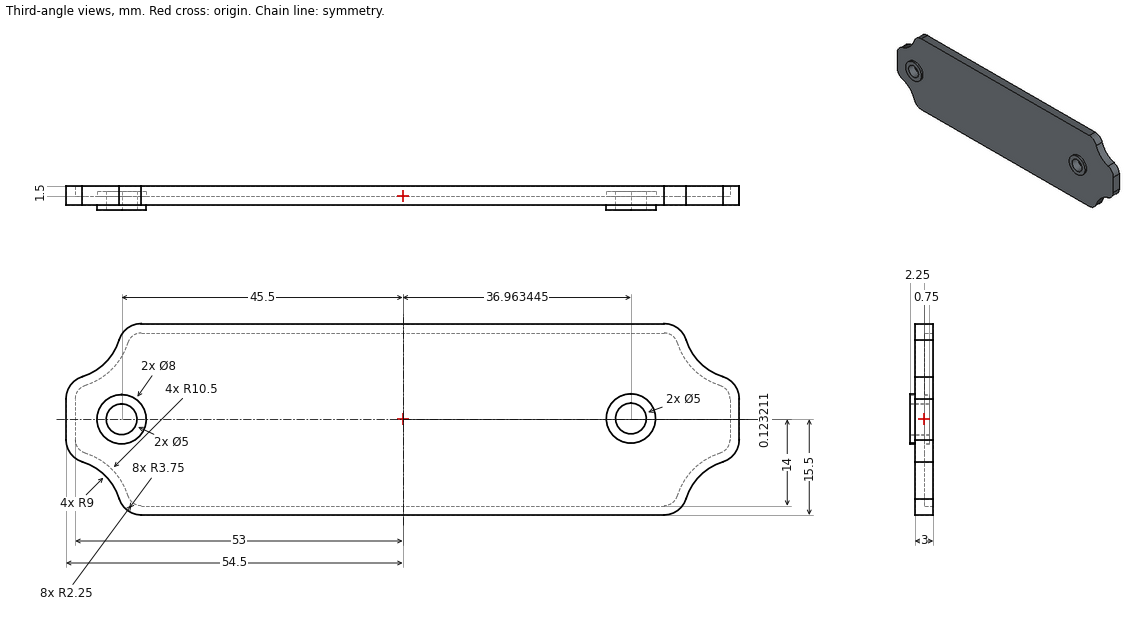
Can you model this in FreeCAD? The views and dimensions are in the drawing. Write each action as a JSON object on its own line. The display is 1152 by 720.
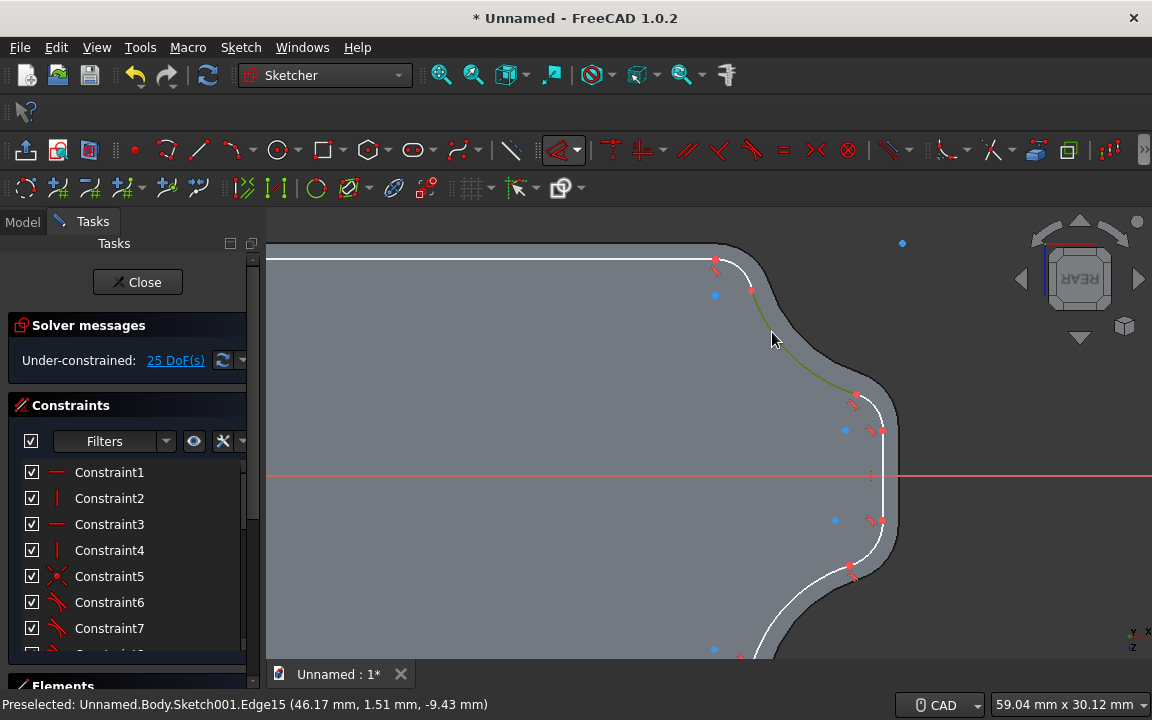
{"action": "left_click", "coordinate": [747, 276]}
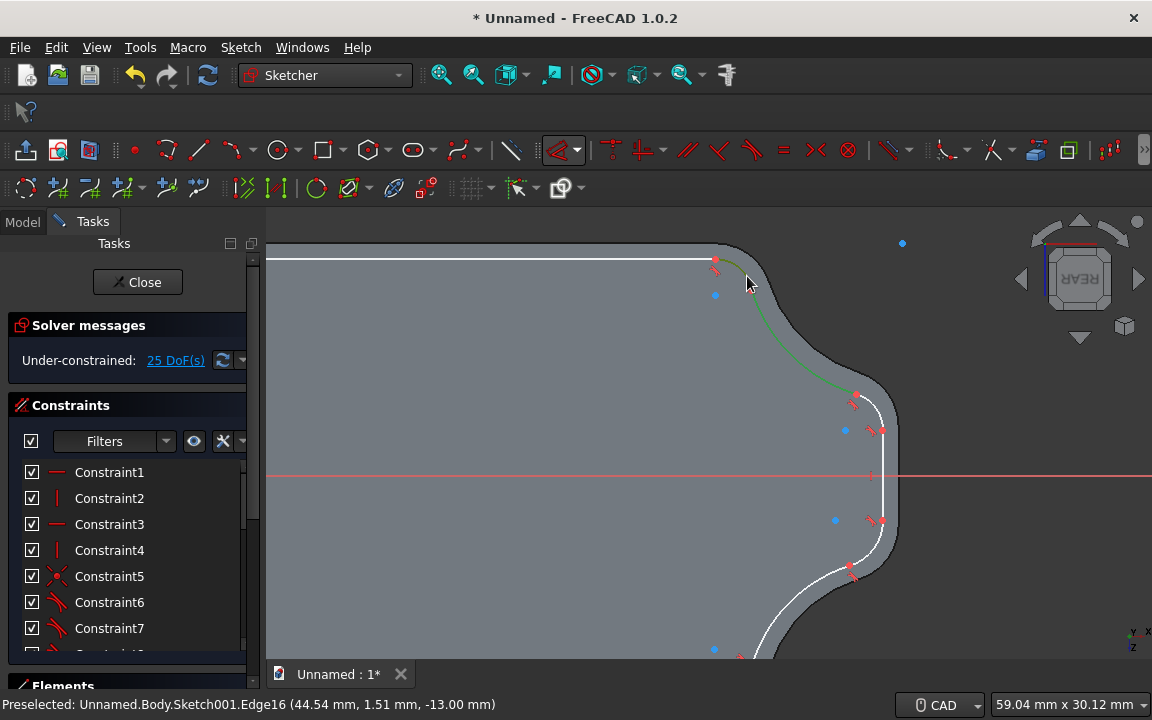
{"action": "left_click", "coordinate": [752, 150]}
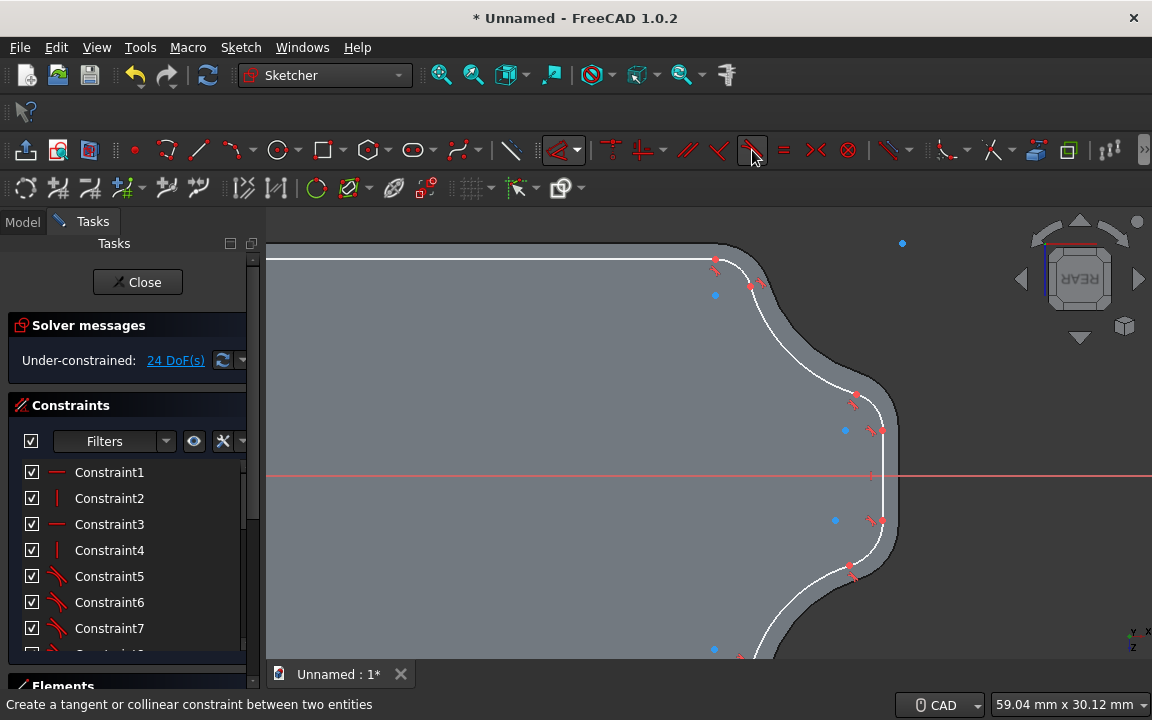
{"action": "scroll", "coordinate": [882, 415], "scroll_direction": "down", "scroll_amount": 6}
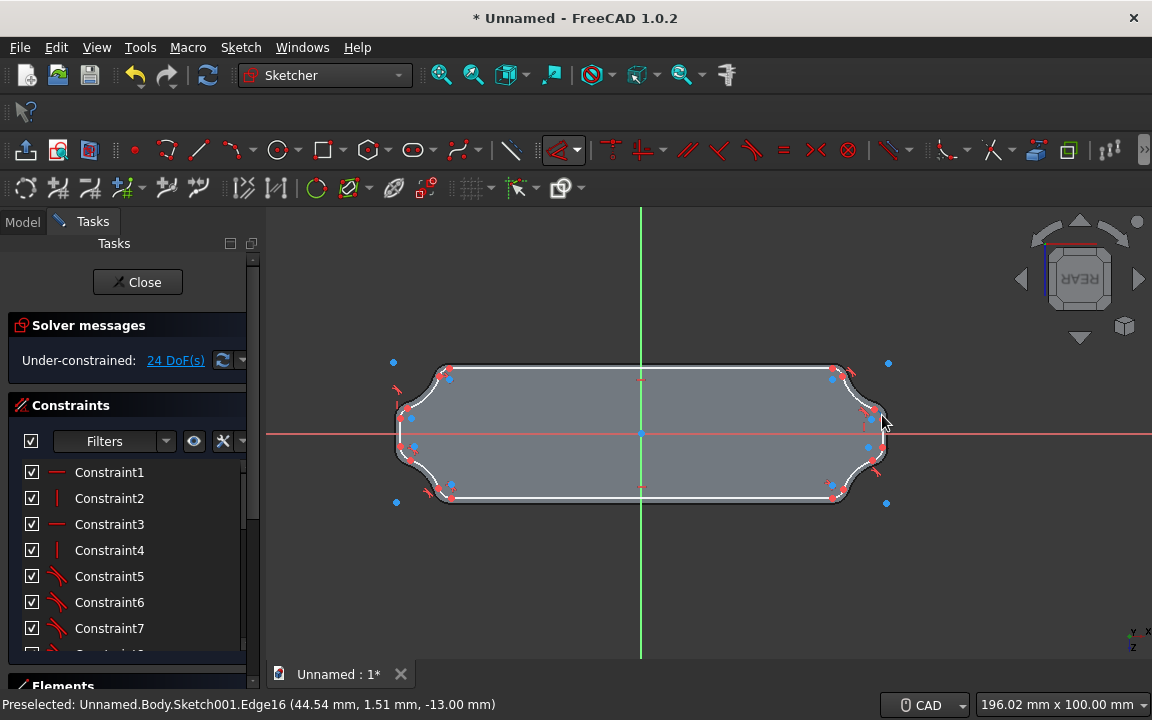
{"action": "scroll", "coordinate": [446, 369], "scroll_direction": "up", "scroll_amount": 7}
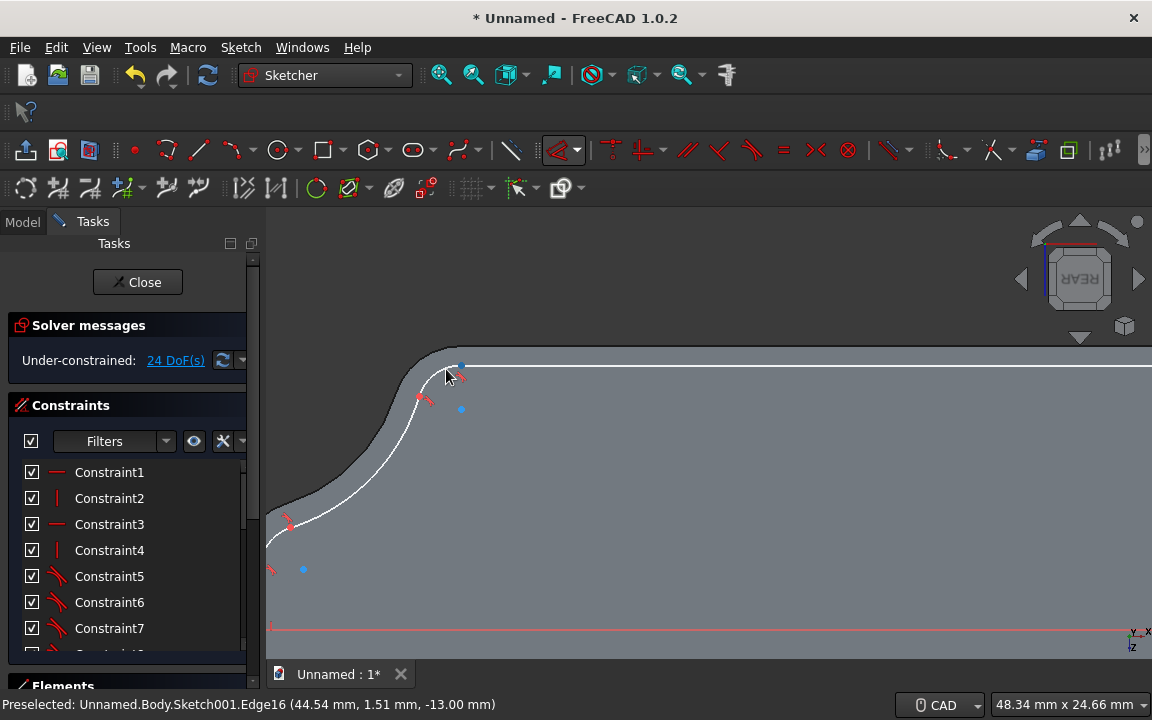
{"action": "left_click", "coordinate": [445, 369]}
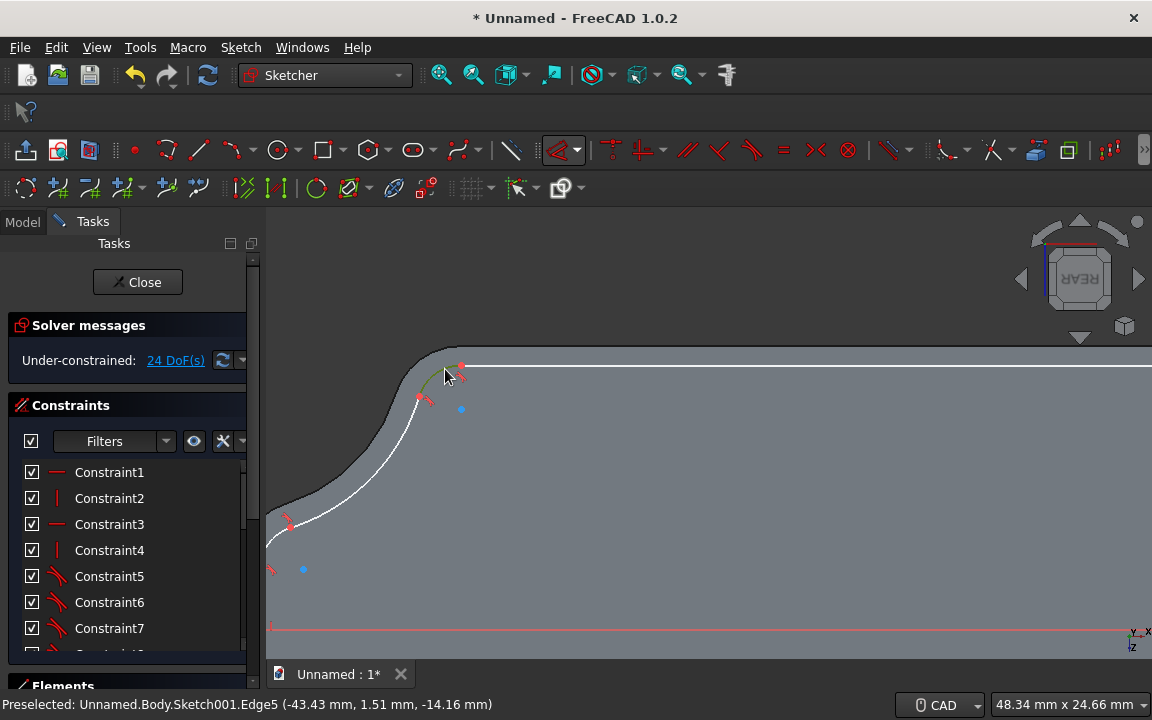
{"action": "scroll", "coordinate": [445, 368], "scroll_direction": "down", "scroll_amount": 7}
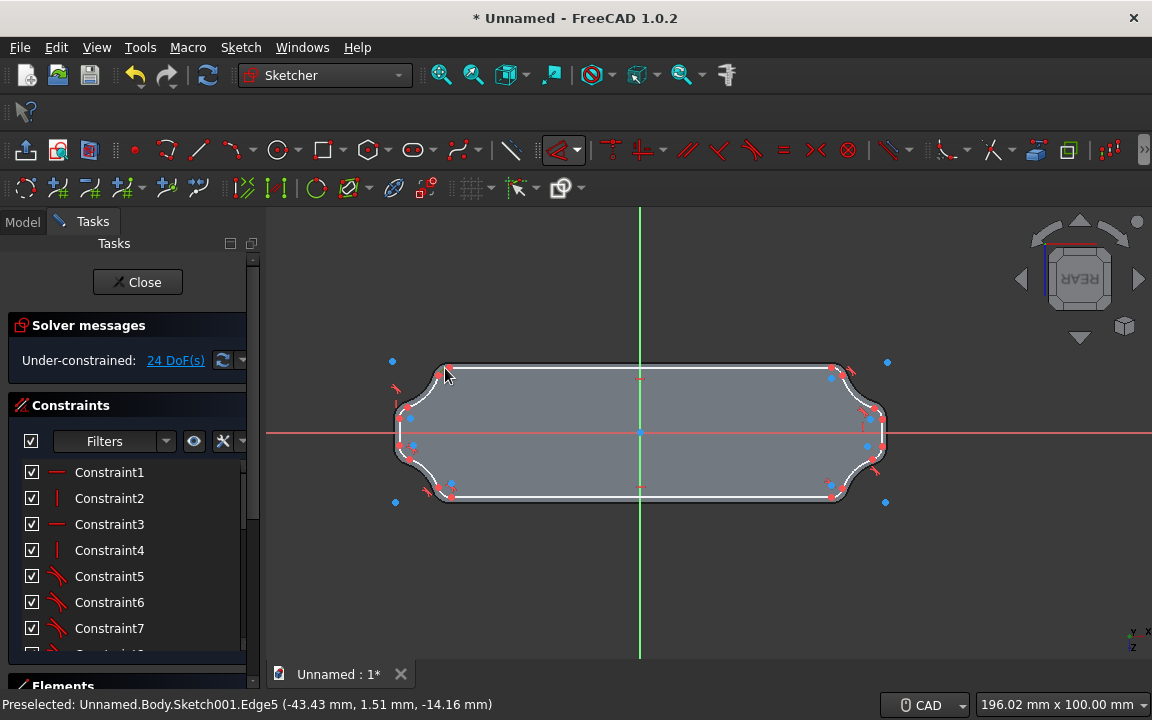
{"action": "scroll", "coordinate": [404, 410], "scroll_direction": "up", "scroll_amount": 7}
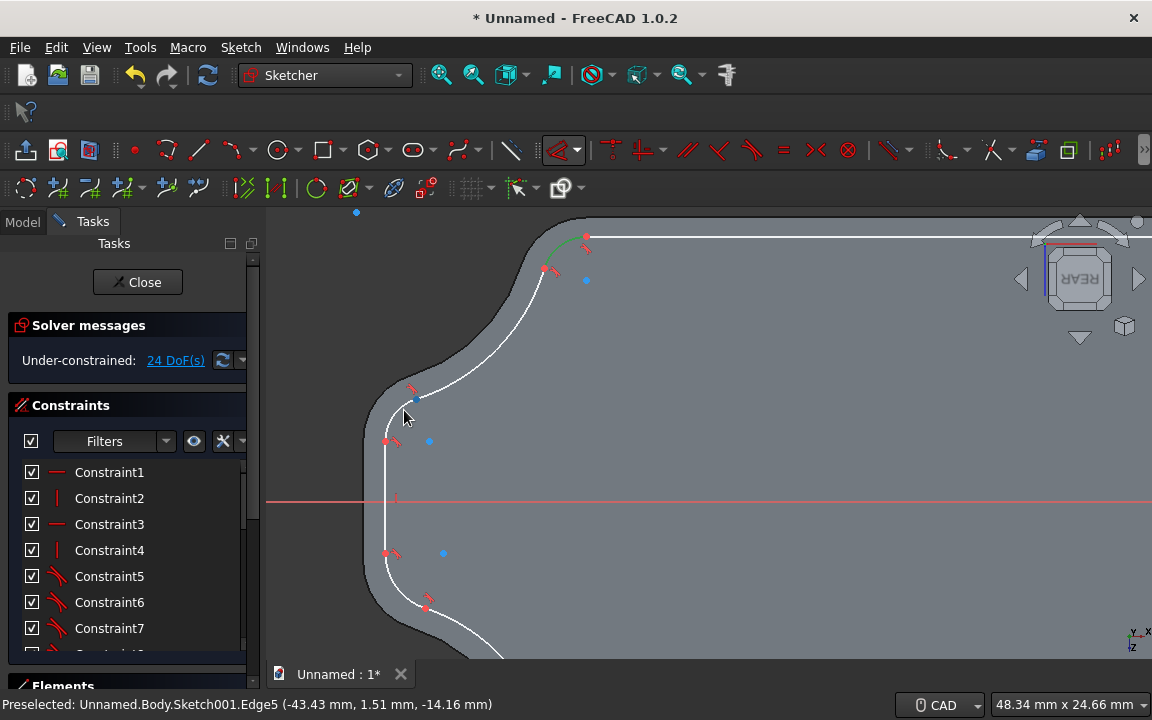
{"action": "left_click", "coordinate": [402, 407]}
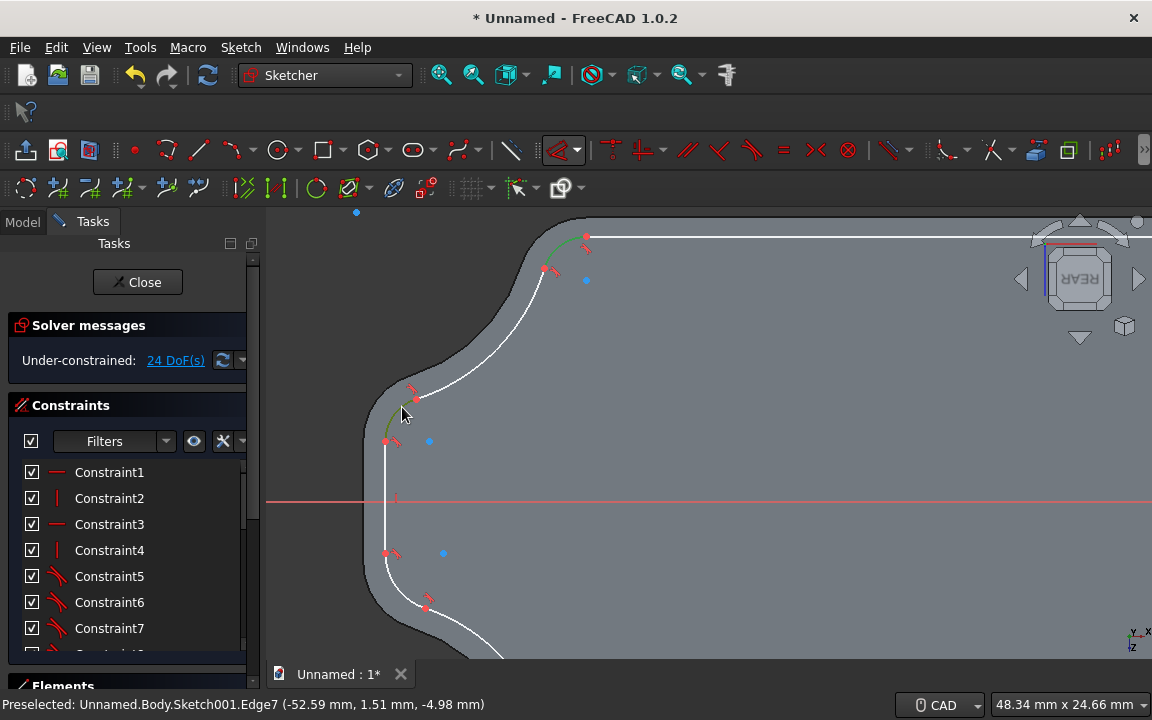
{"action": "left_click", "coordinate": [390, 574]}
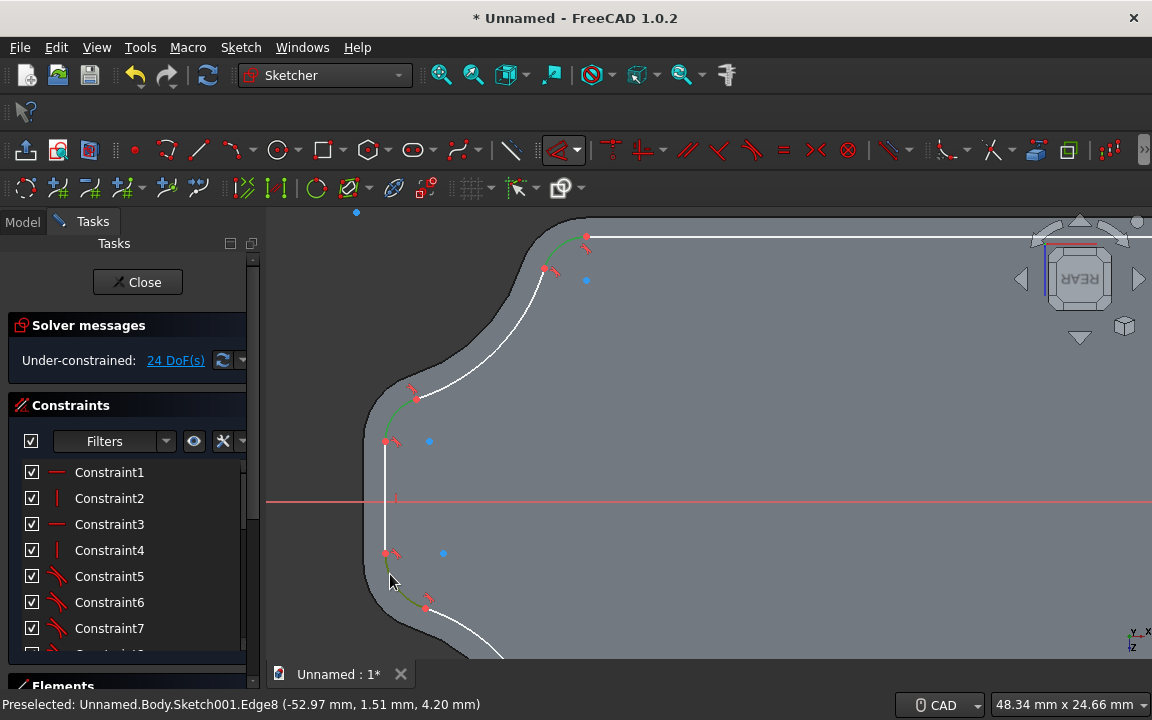
{"action": "scroll", "coordinate": [404, 411], "scroll_direction": "down", "scroll_amount": 7}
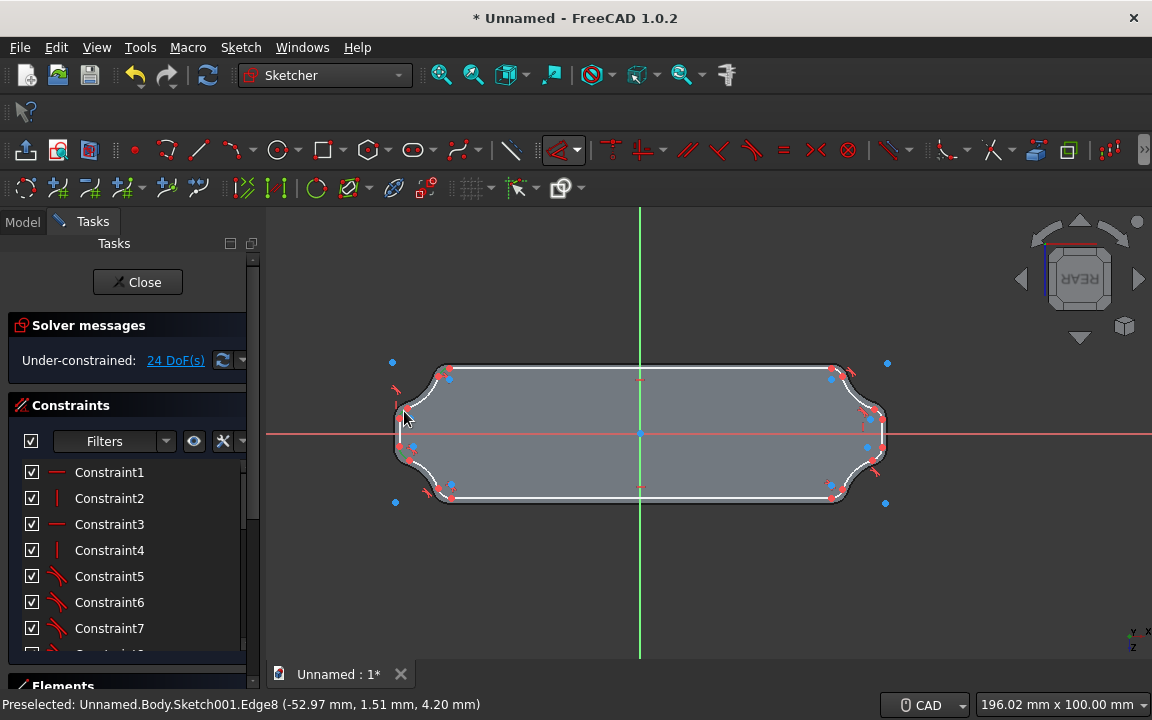
{"action": "scroll", "coordinate": [441, 493], "scroll_direction": "up", "scroll_amount": 5}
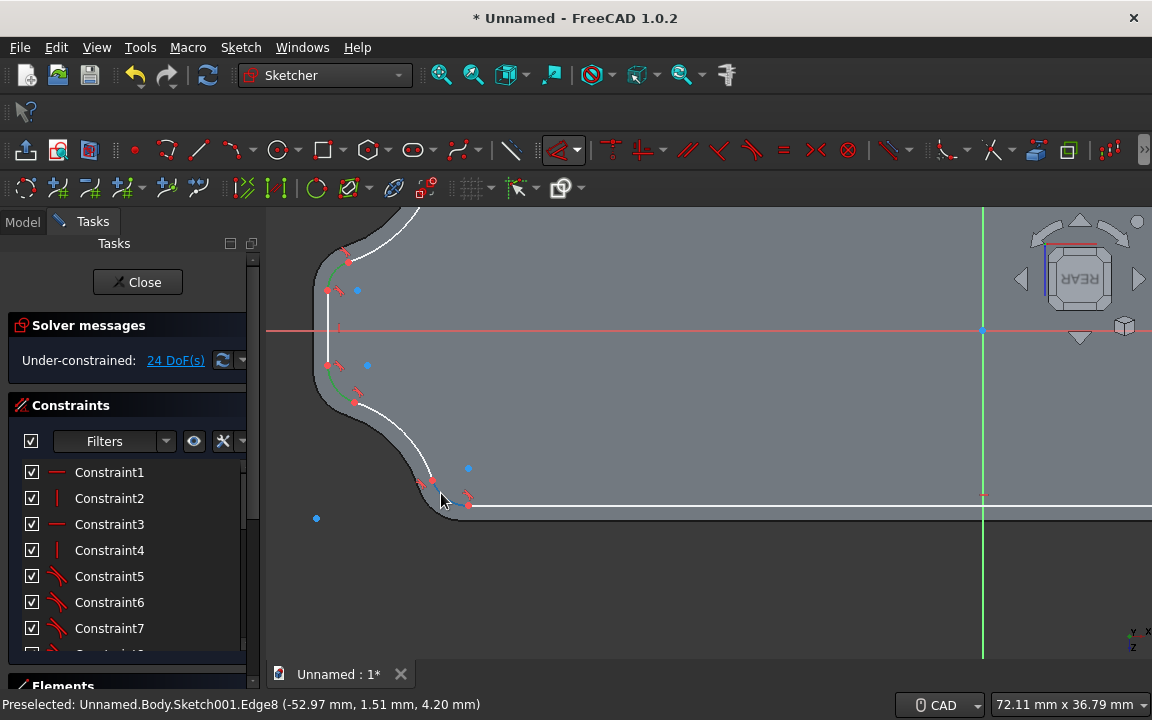
{"action": "left_click", "coordinate": [439, 492]}